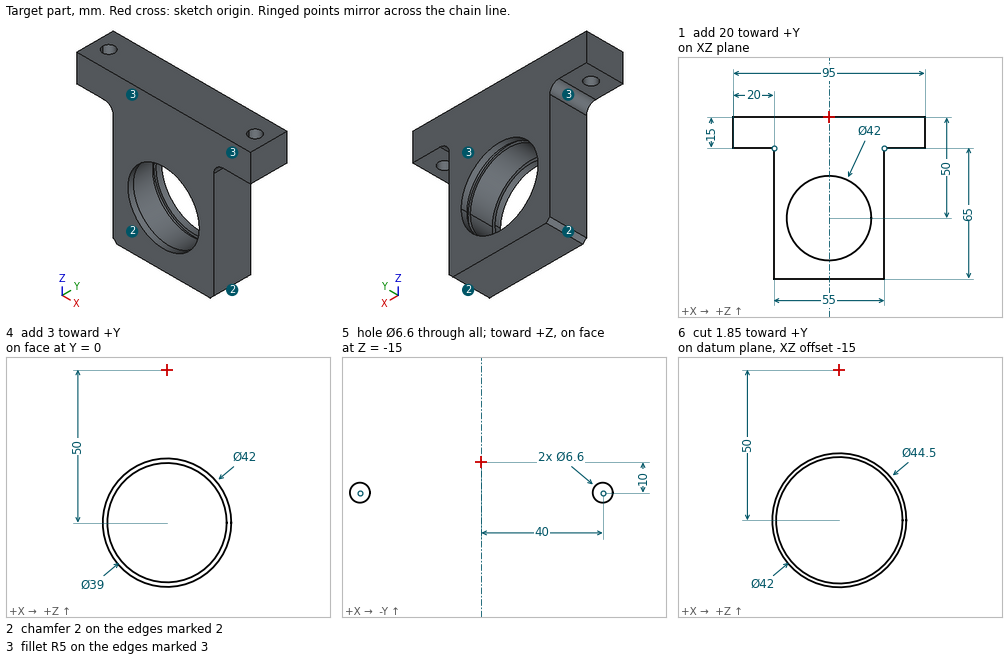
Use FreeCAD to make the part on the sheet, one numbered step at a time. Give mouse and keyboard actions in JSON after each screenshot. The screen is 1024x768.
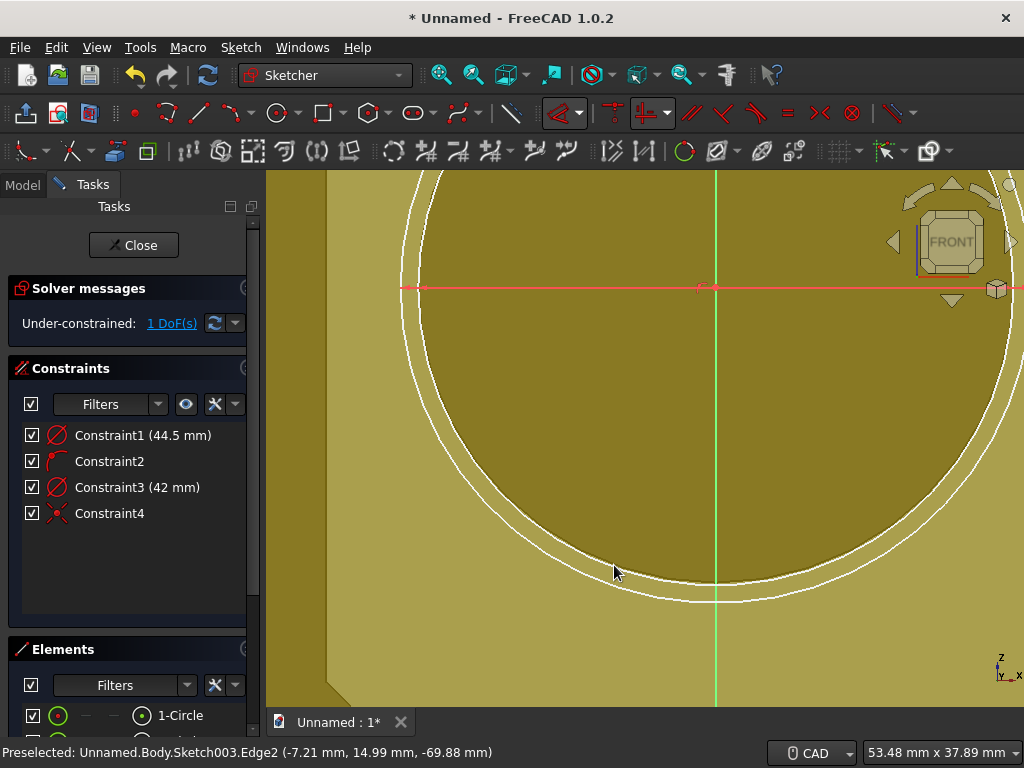
{"action": "left_click", "coordinate": [716, 288]}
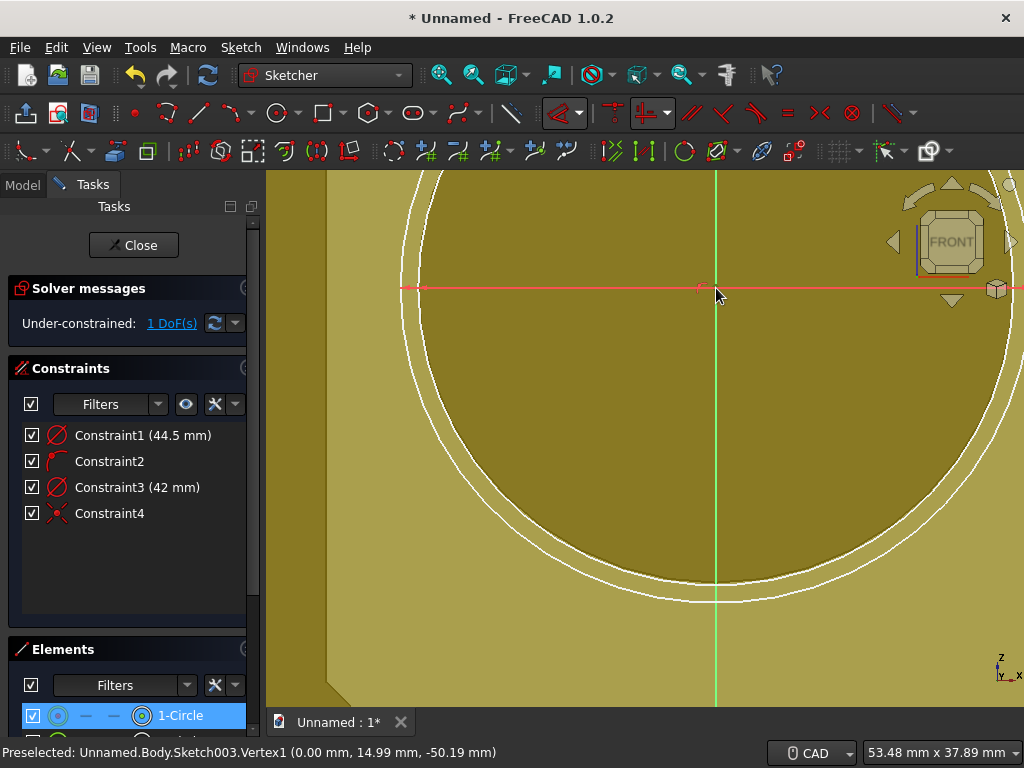
{"action": "key", "text": "i"}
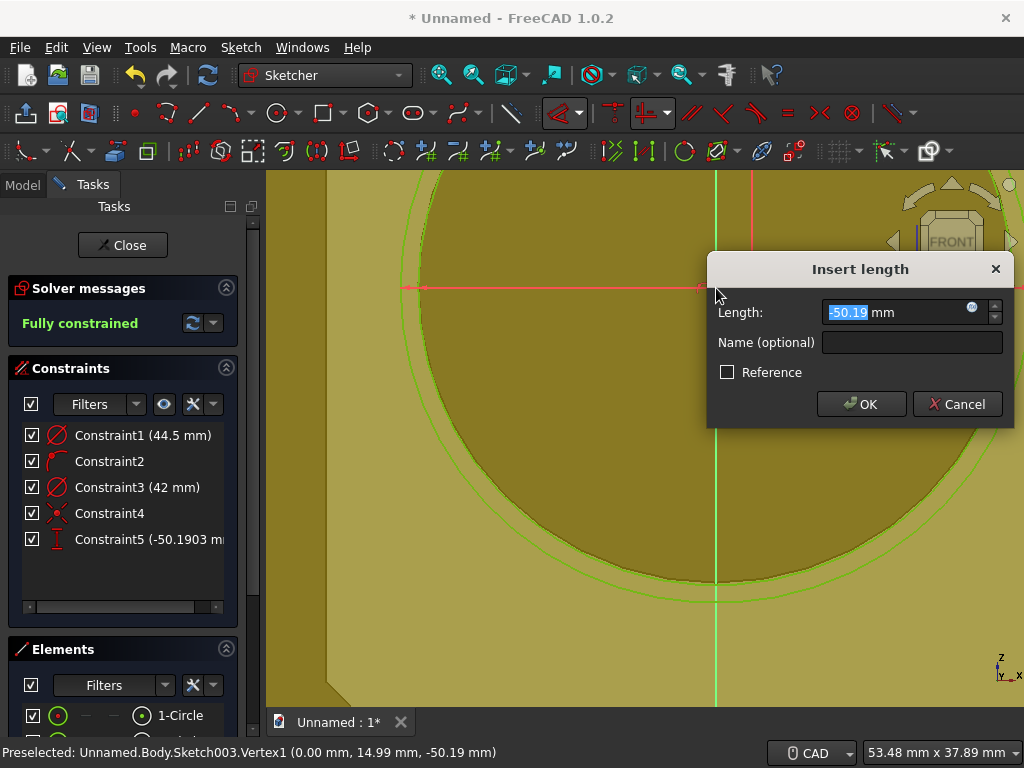
{"action": "type", "text": "-50"}
{"action": "key", "text": "Return"}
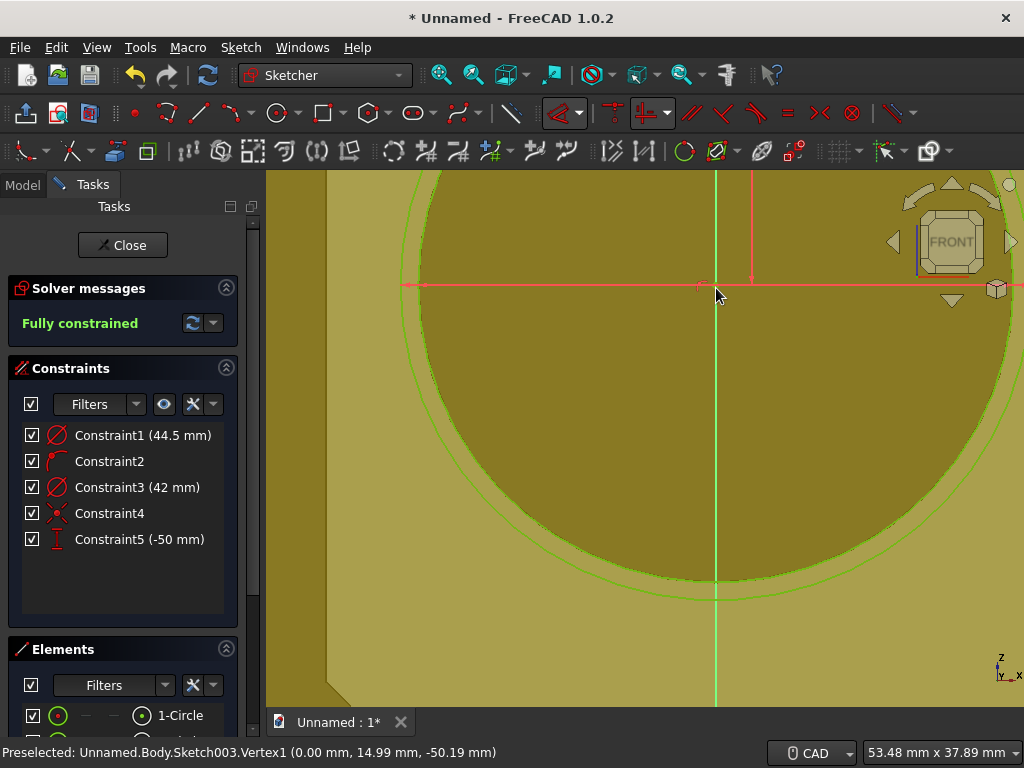
{"action": "left_click", "coordinate": [123, 245]}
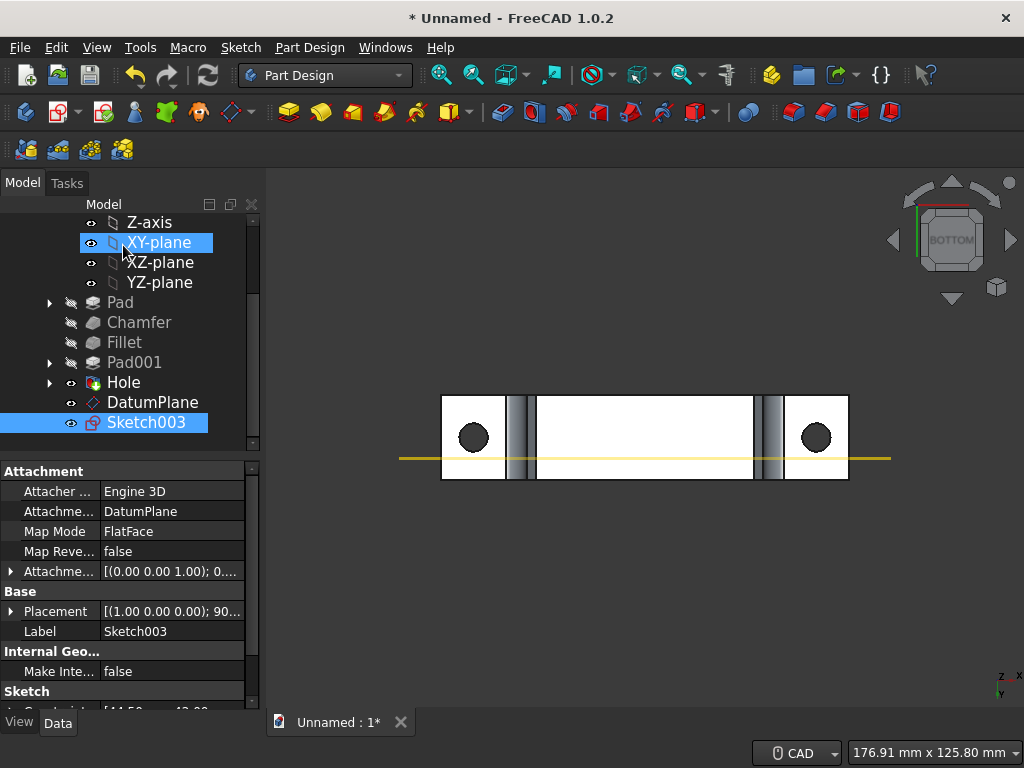
{"action": "left_click", "coordinate": [504, 112]}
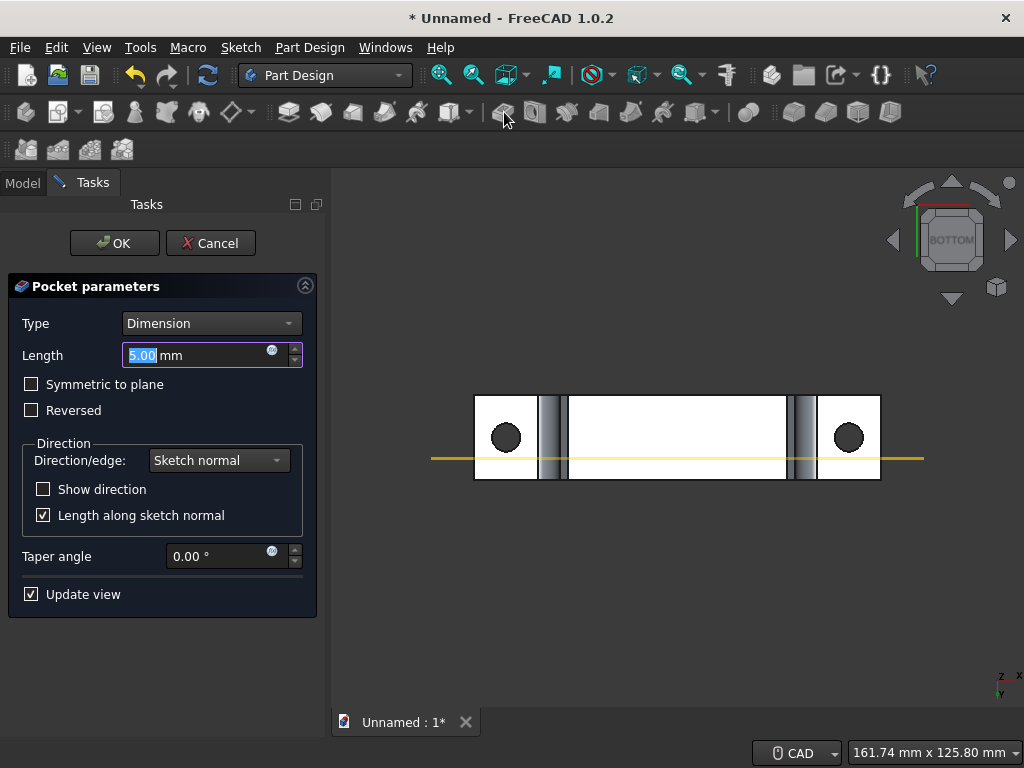
{"action": "type", "text": "1.85"}
{"action": "key", "text": "Tab"}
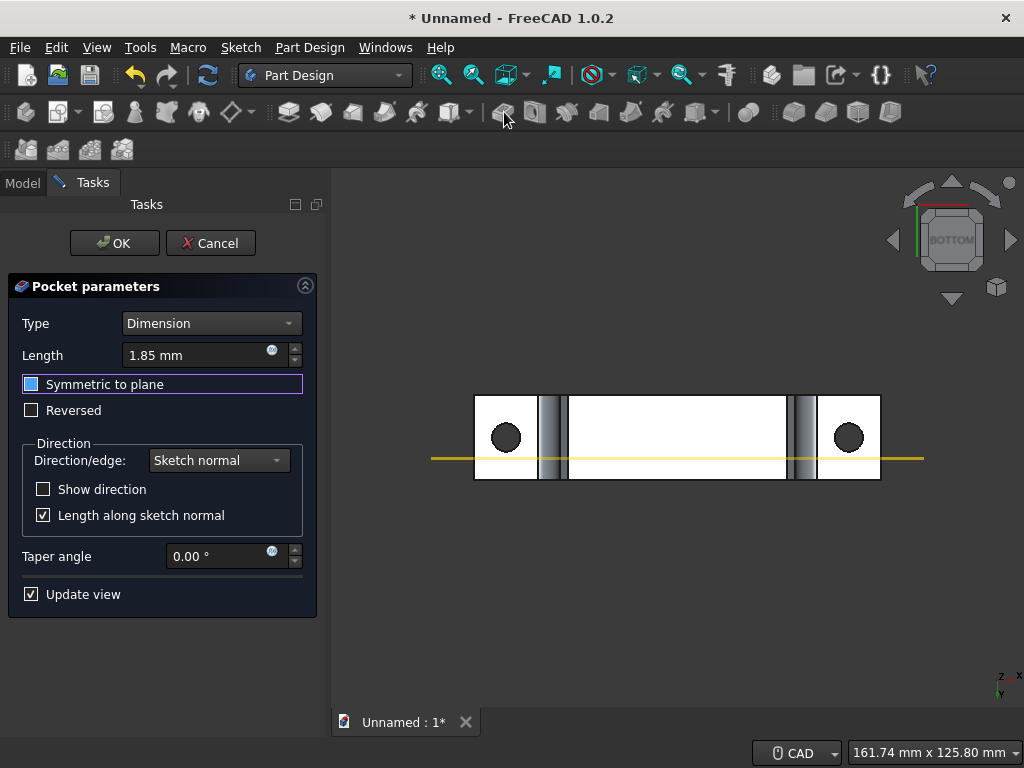
{"action": "left_click", "coordinate": [115, 243]}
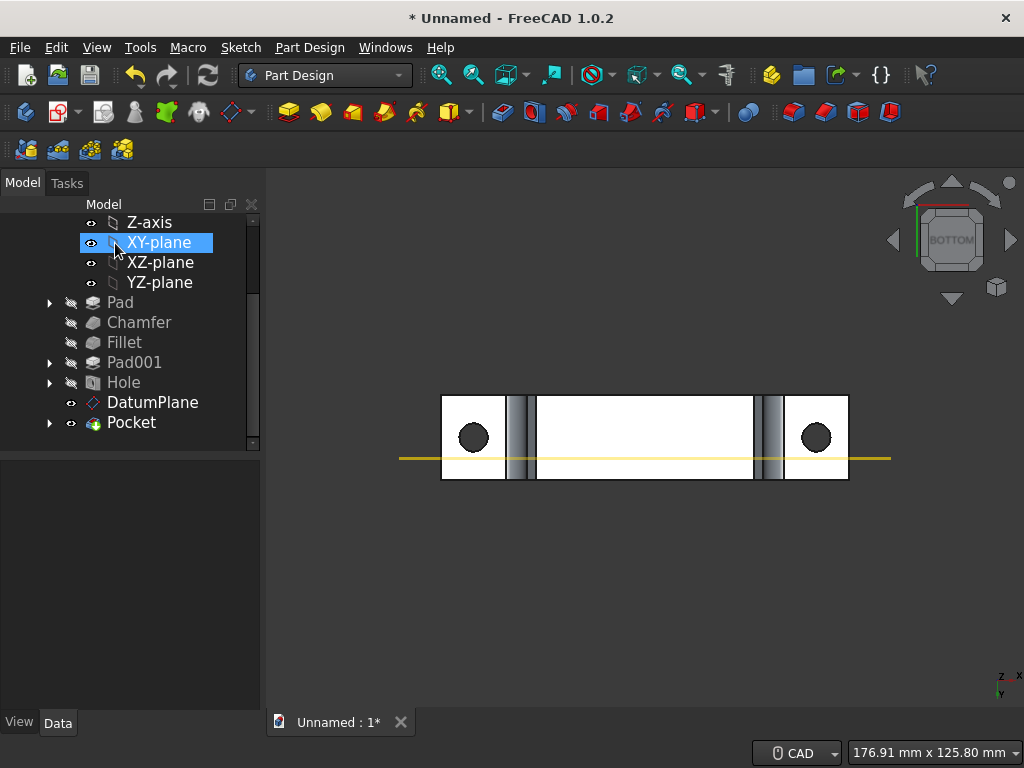
{"action": "left_click", "coordinate": [116, 403]}
{"action": "key", "text": "space"}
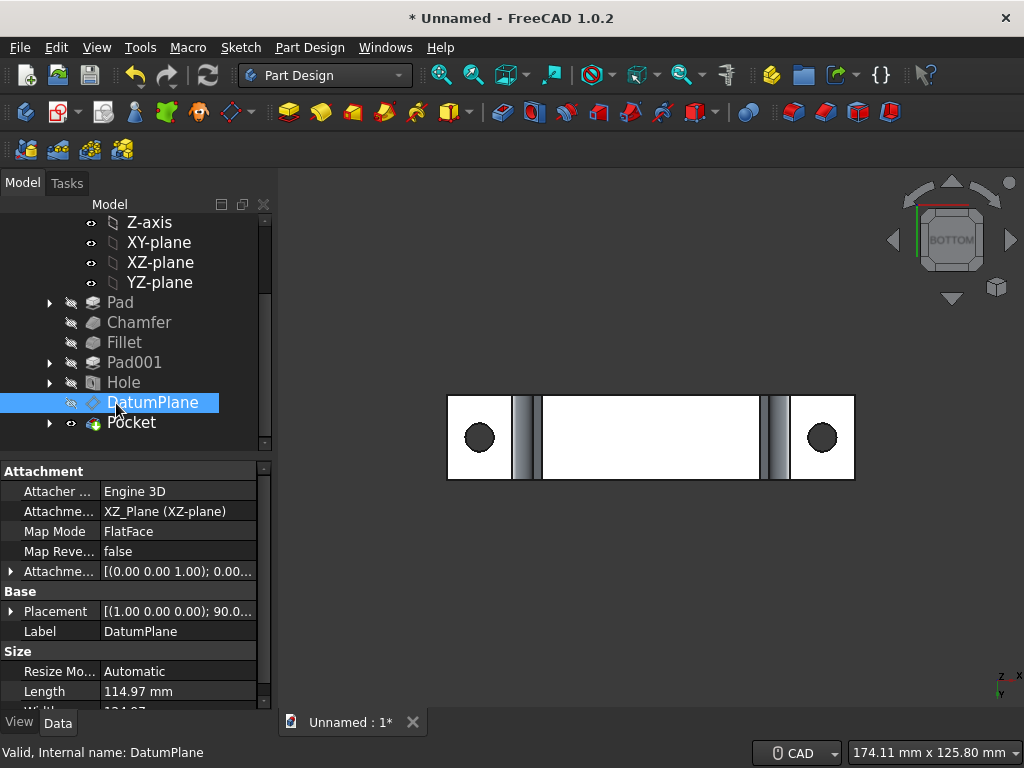
{"action": "key", "text": "0"}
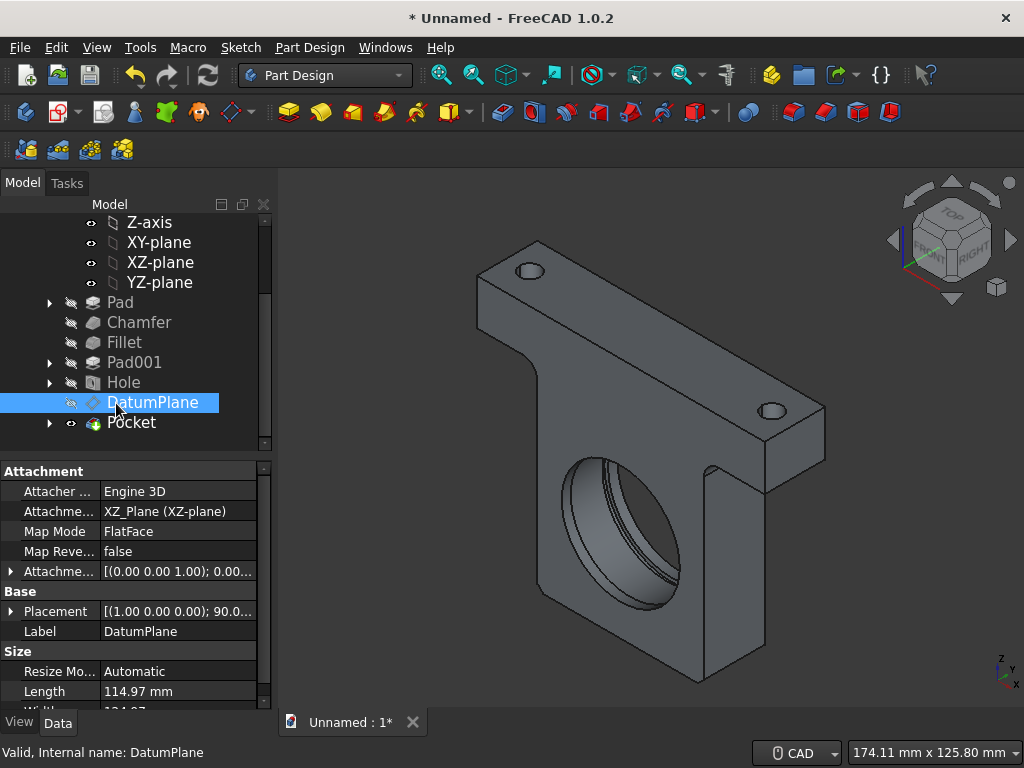
{"action": "left_click", "coordinate": [442, 76]}